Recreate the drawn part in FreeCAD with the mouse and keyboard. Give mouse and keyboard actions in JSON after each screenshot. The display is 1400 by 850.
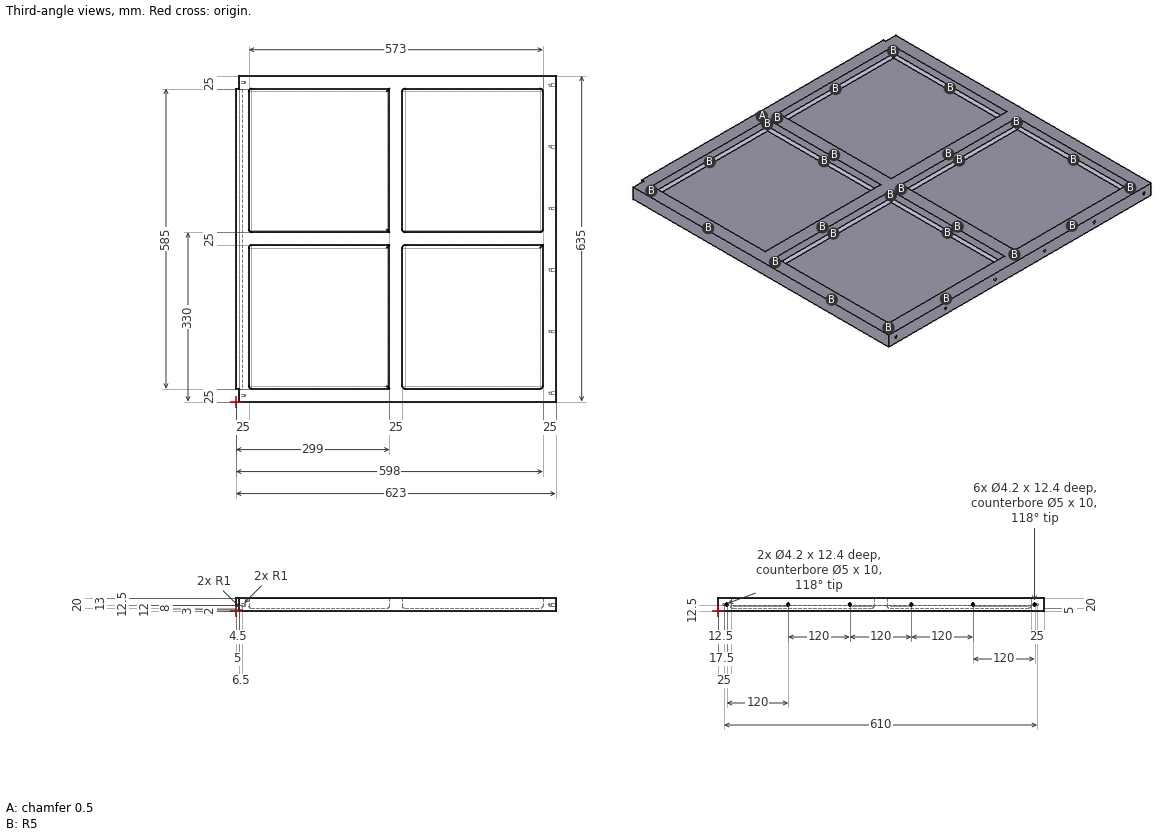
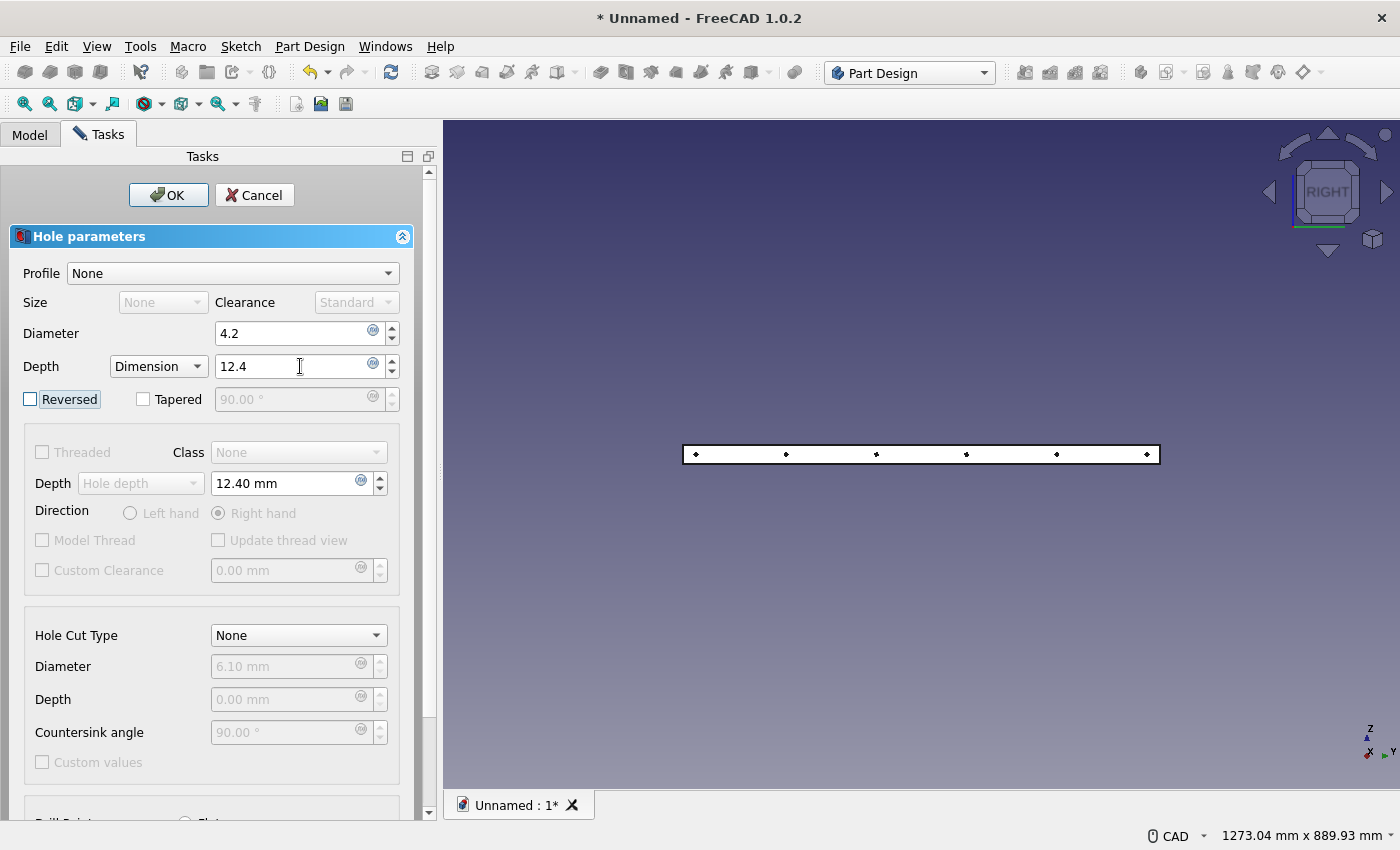
{"action": "left_click", "coordinate": [300, 636]}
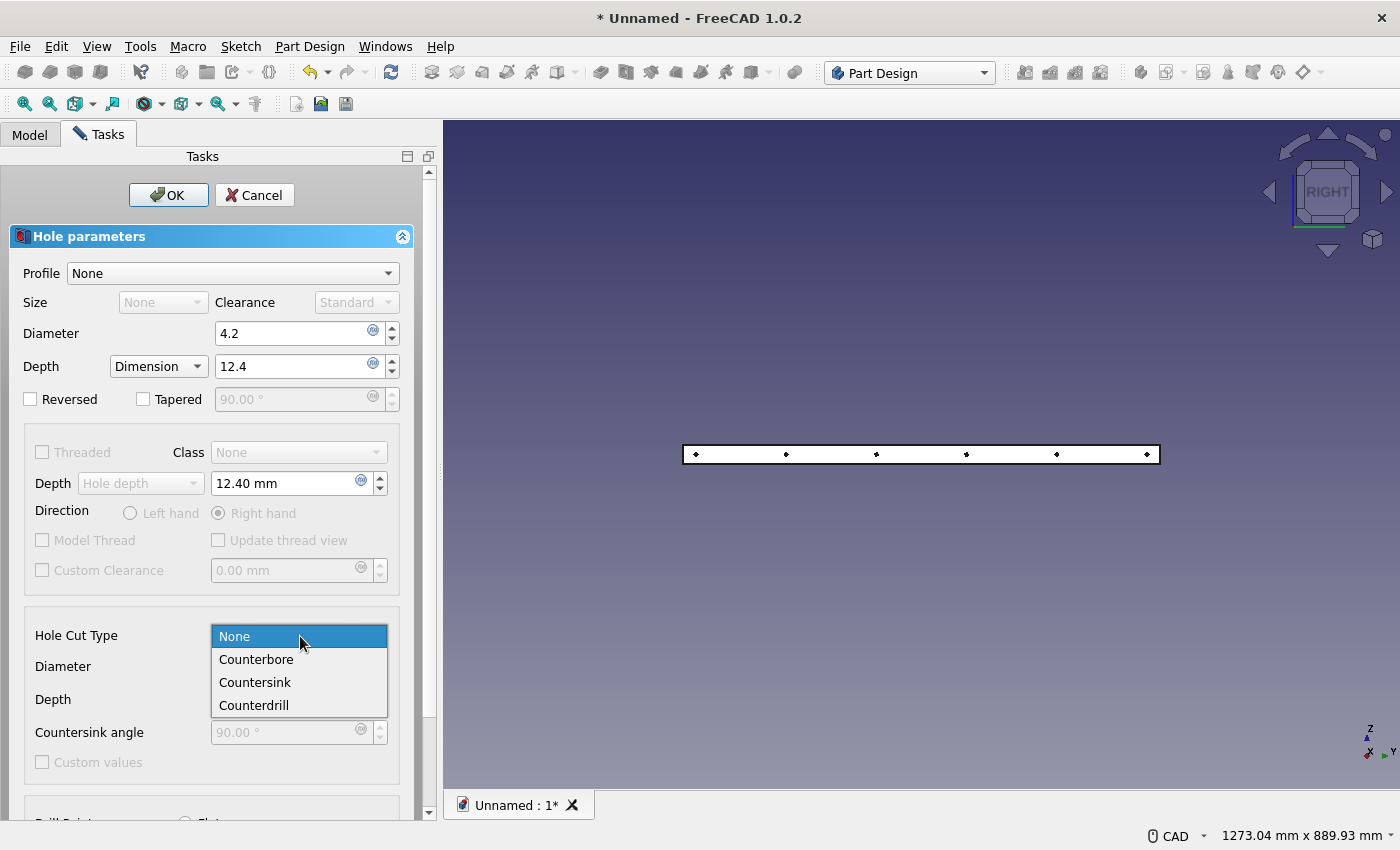
{"action": "left_click", "coordinate": [298, 660]}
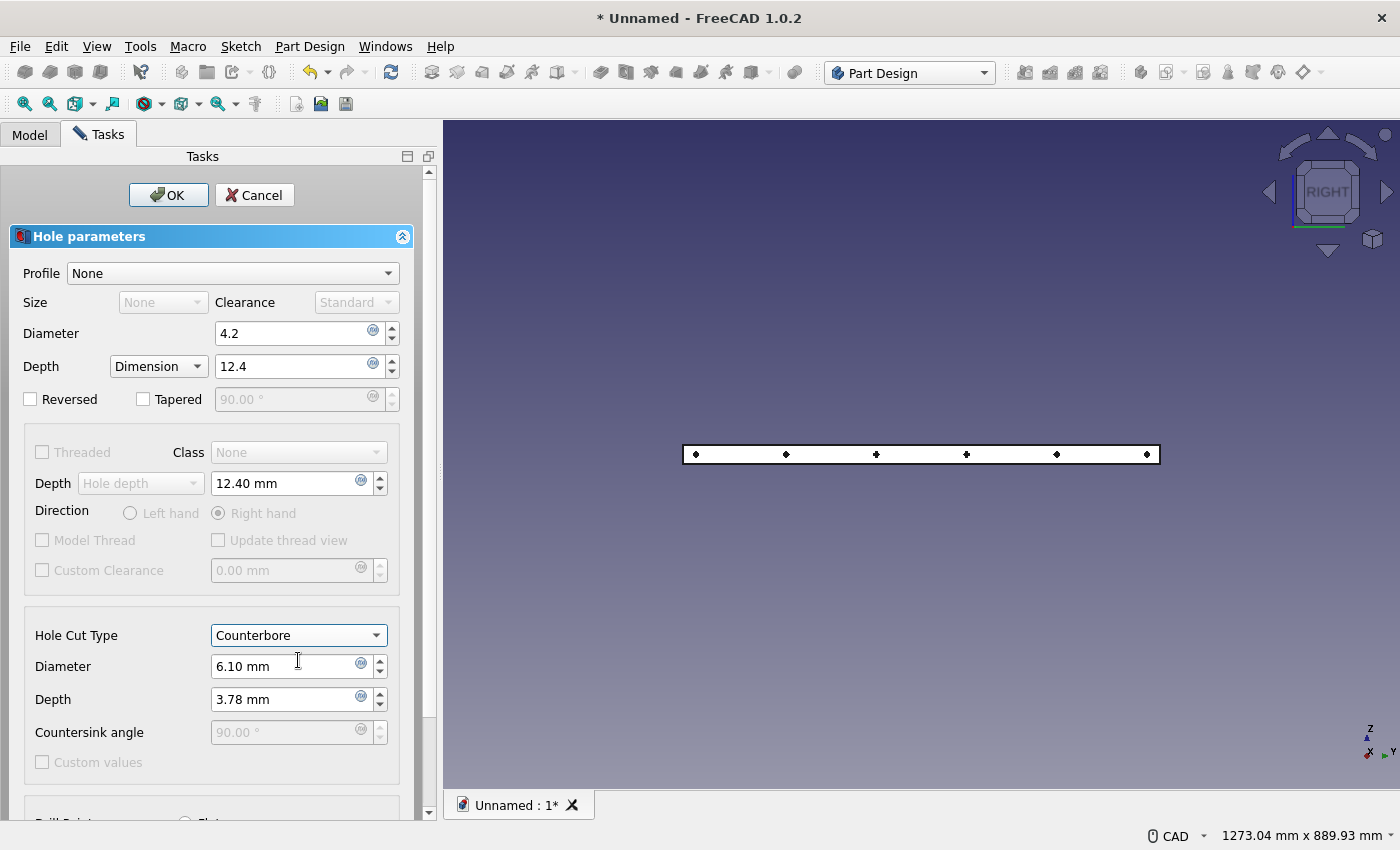
{"action": "triple_click", "coordinate": [292, 666]}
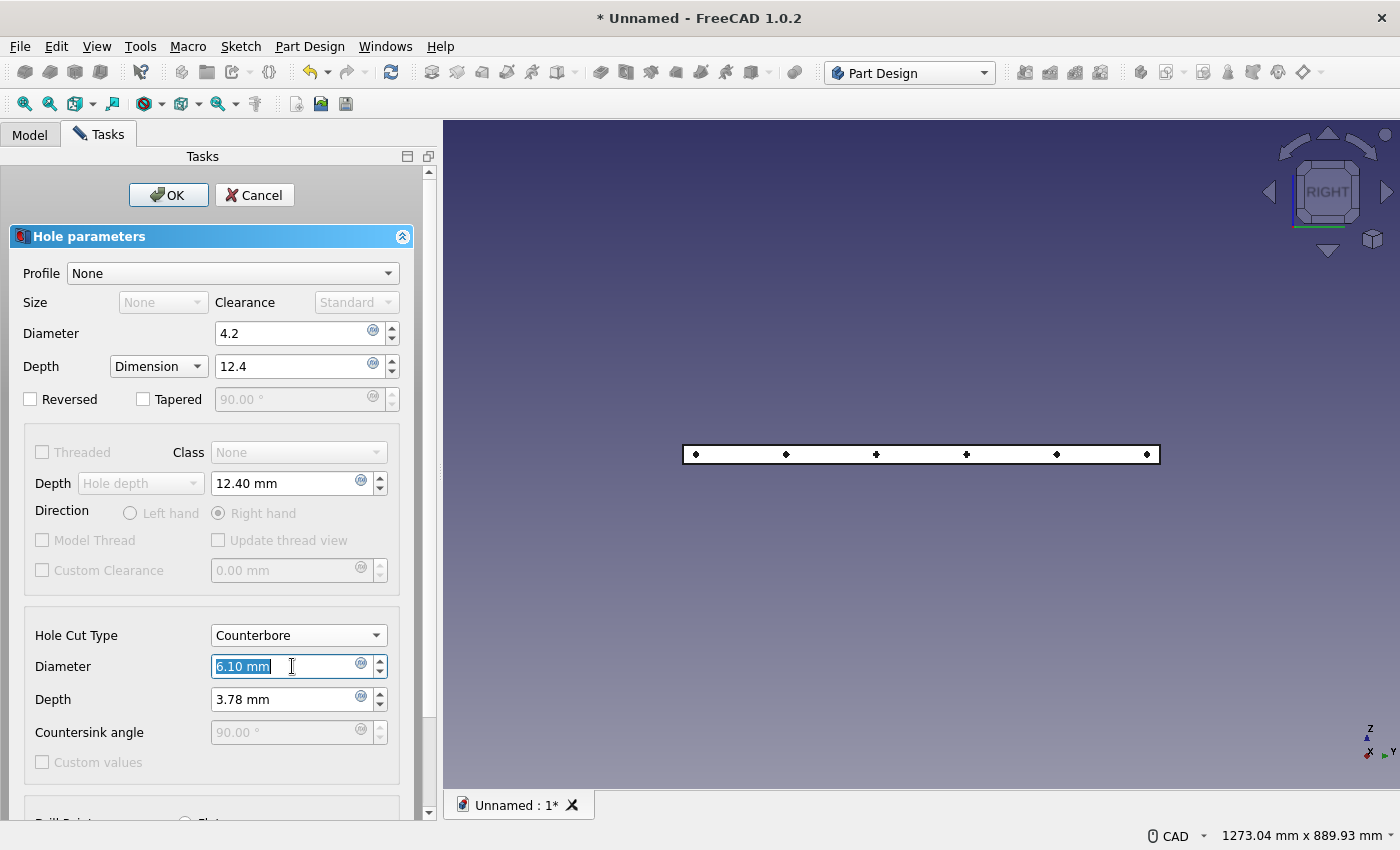
{"action": "type", "text": "5"}
{"action": "key", "text": "Tab"}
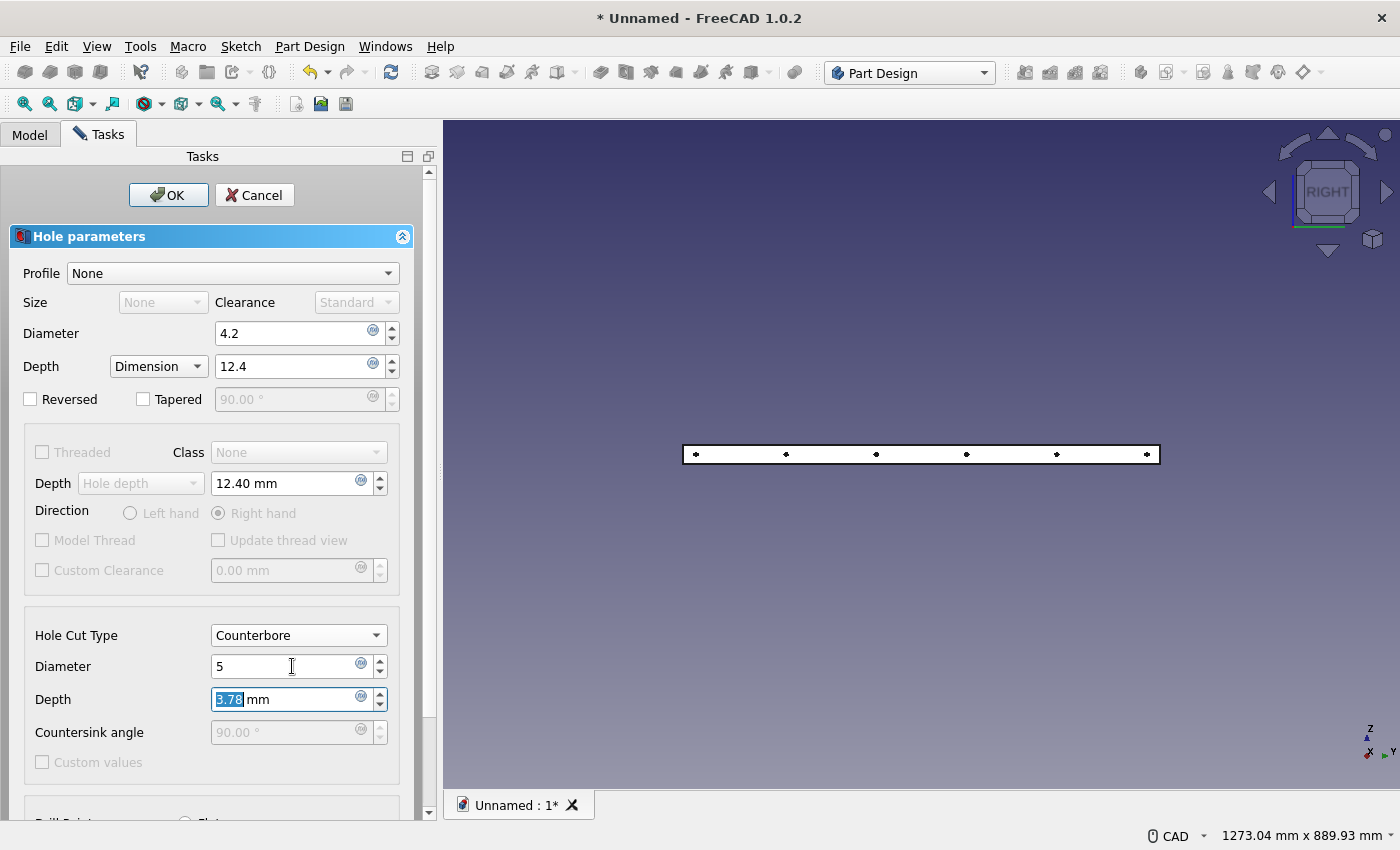
{"action": "type", "text": "10"}
{"action": "key", "text": "Tab"}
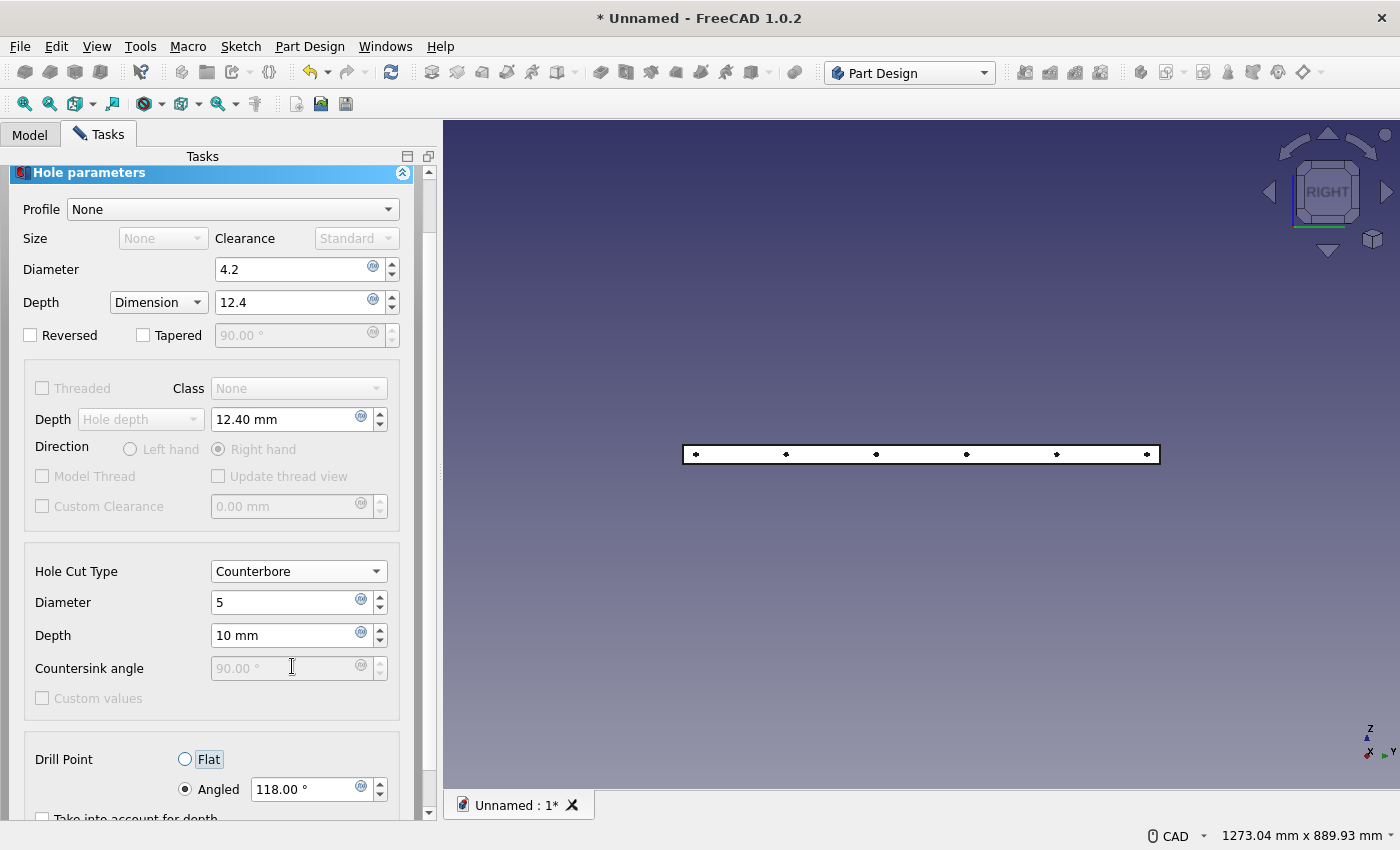
{"action": "scroll", "coordinate": [429, 493], "scroll_direction": "up", "scroll_amount": 2}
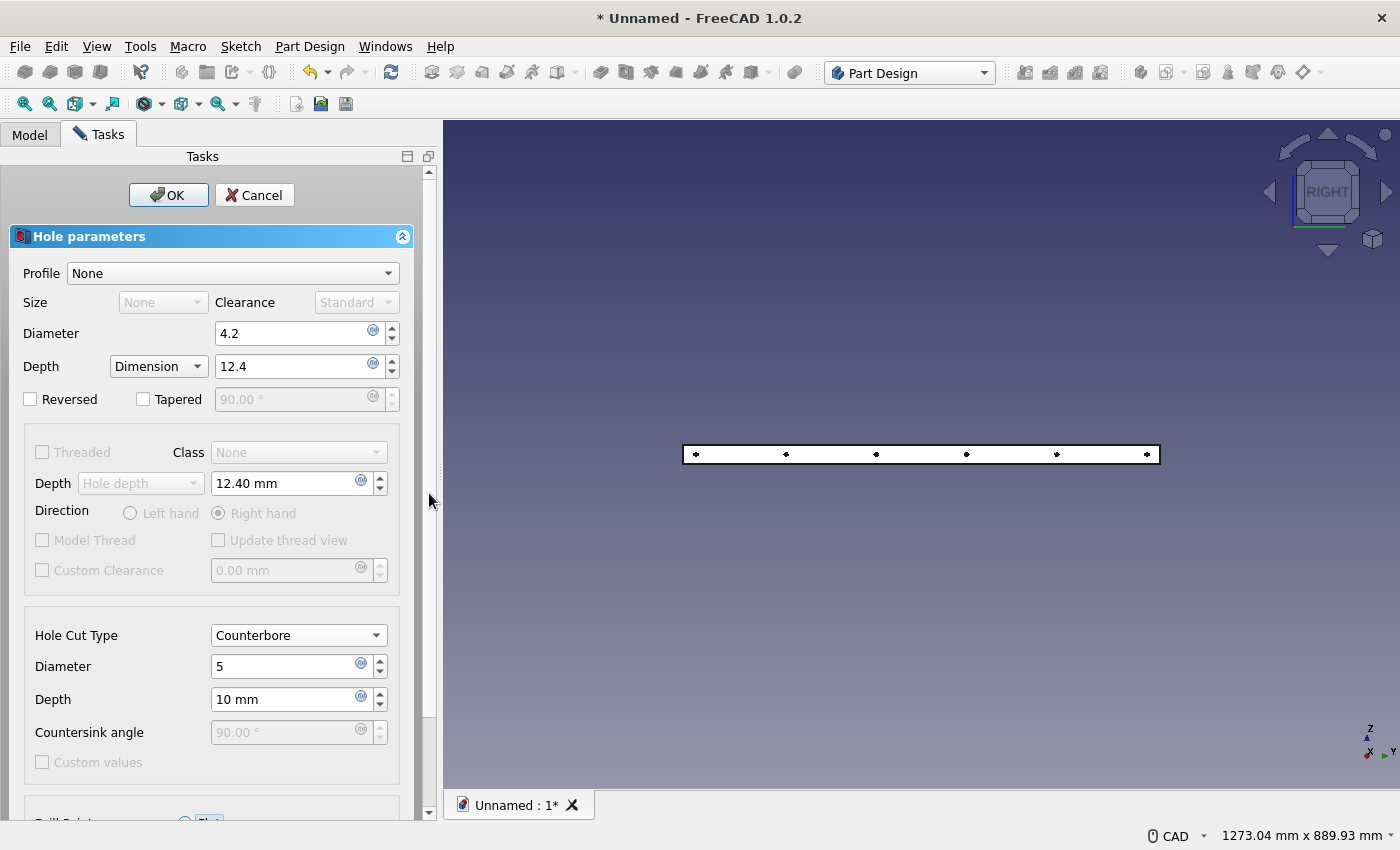
{"action": "left_click", "coordinate": [169, 195]}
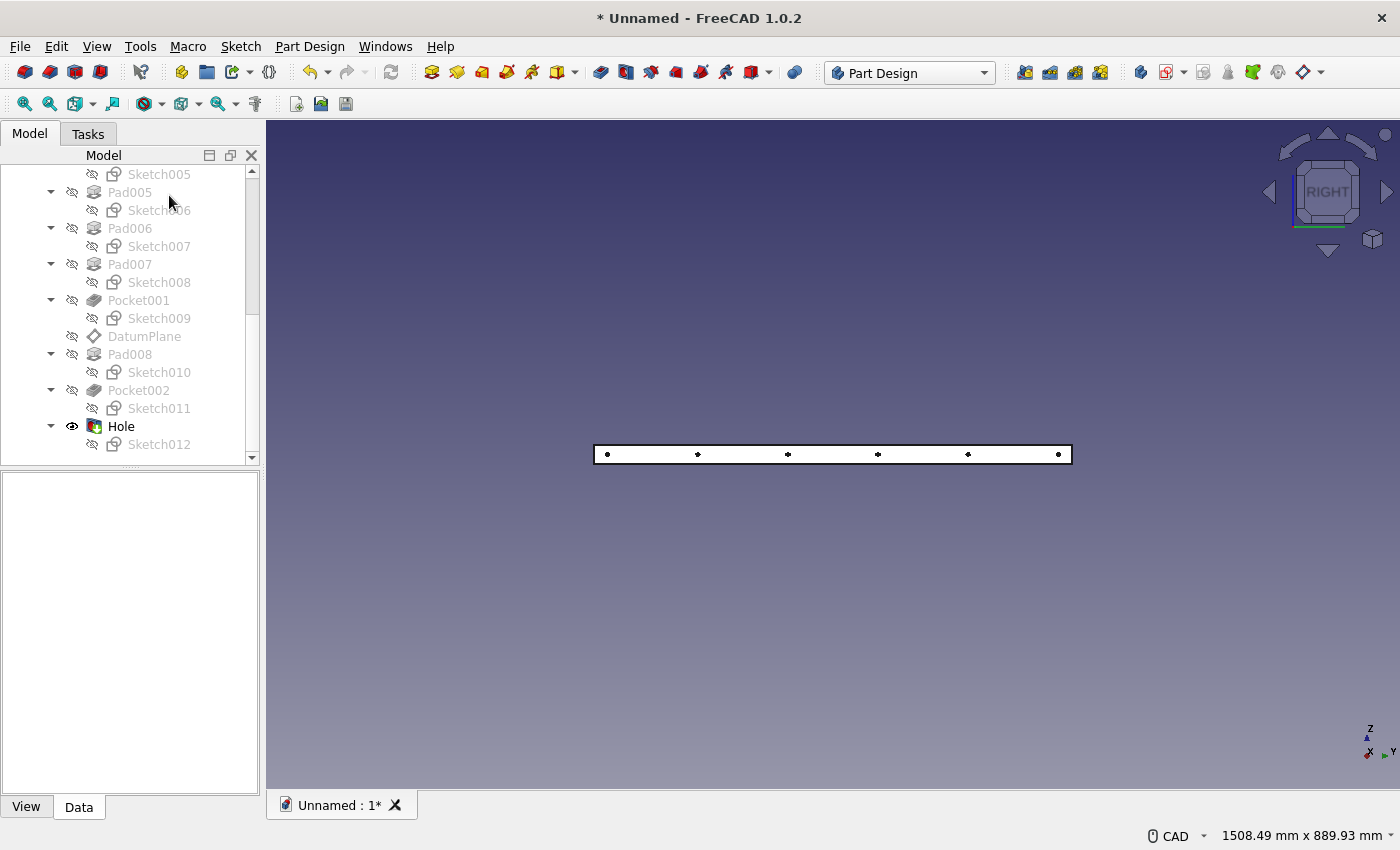
{"action": "left_click", "coordinate": [25, 104]}